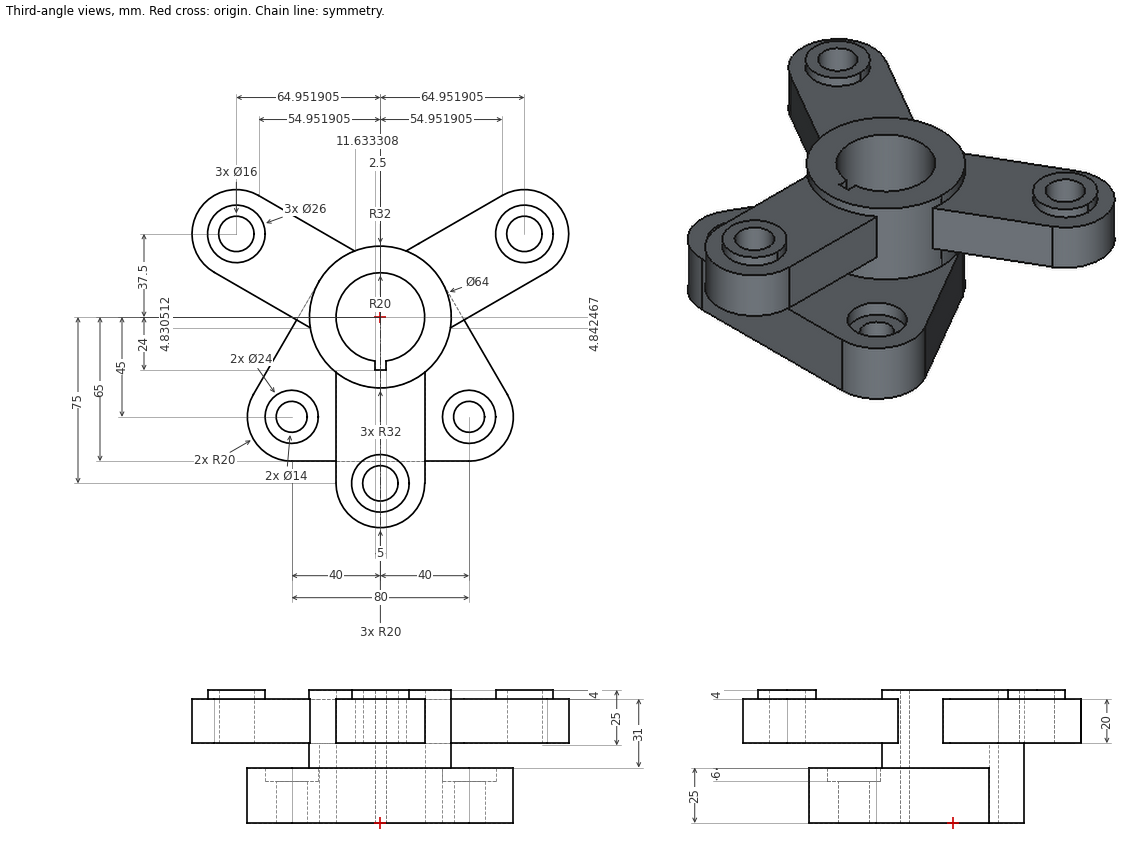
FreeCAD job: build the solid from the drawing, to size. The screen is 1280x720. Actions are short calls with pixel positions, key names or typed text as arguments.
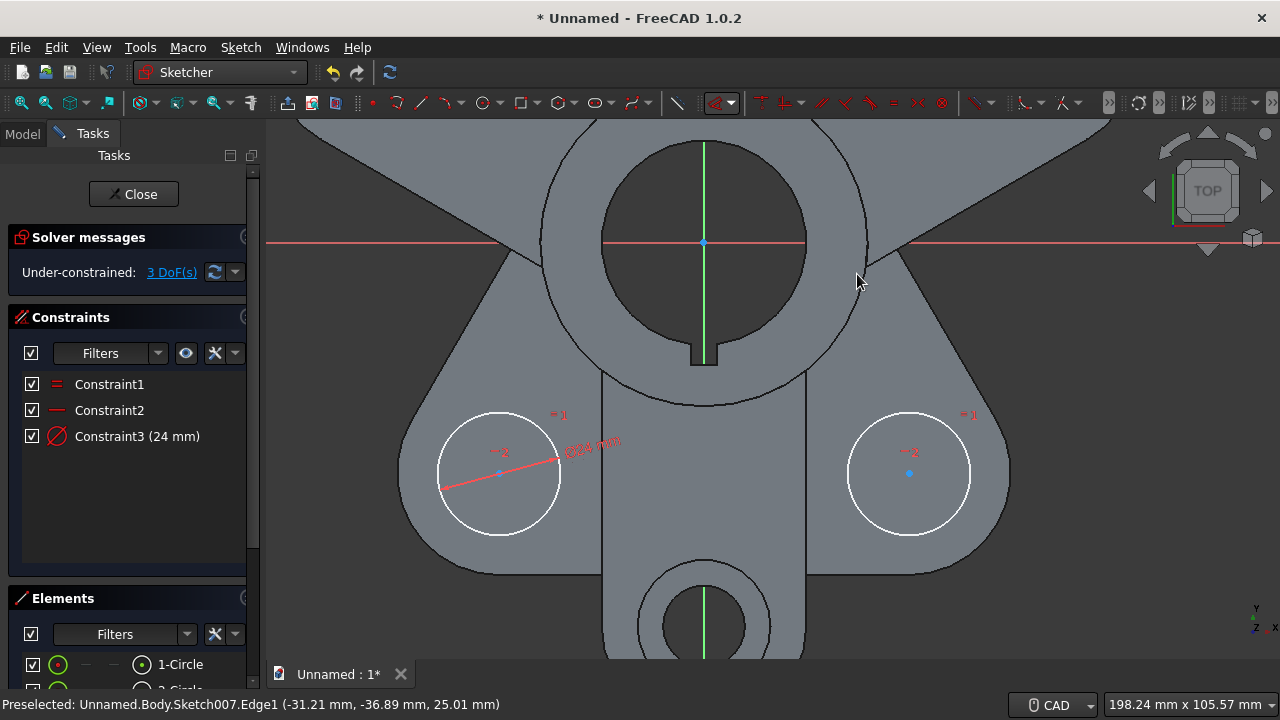
click(499, 474)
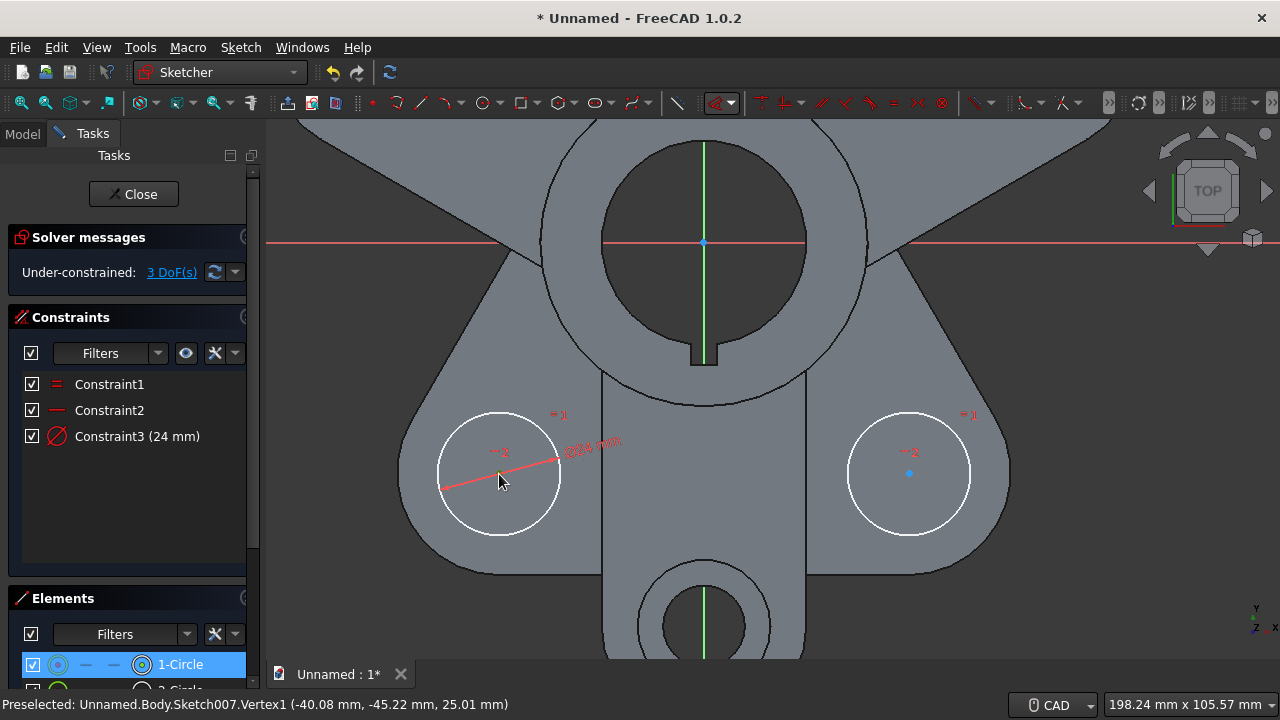
key(l)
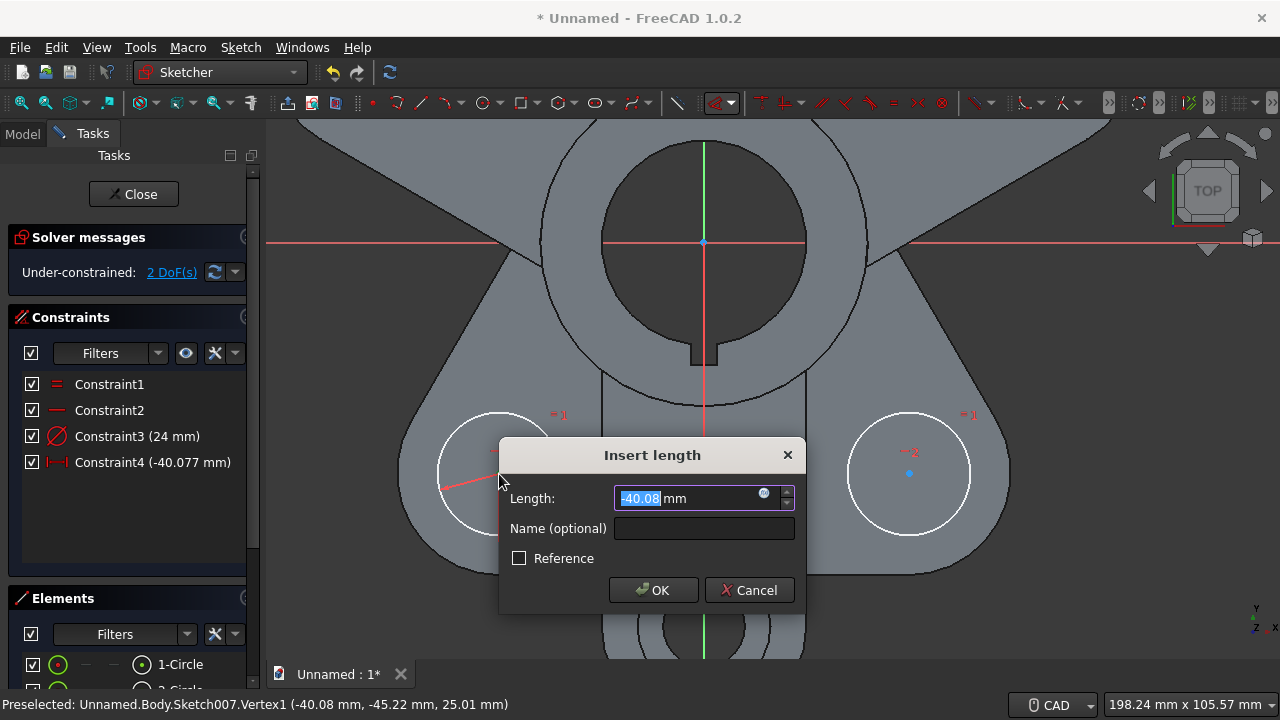
text(-40)
key(Return)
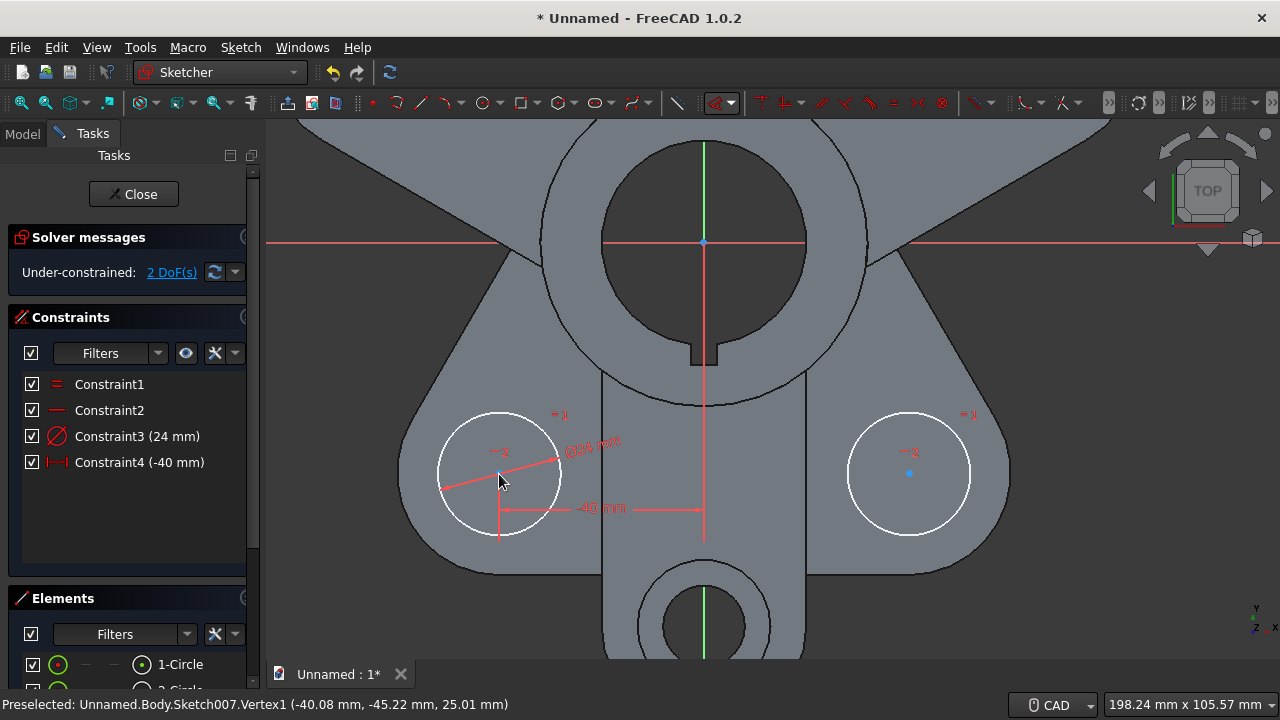
click(499, 474)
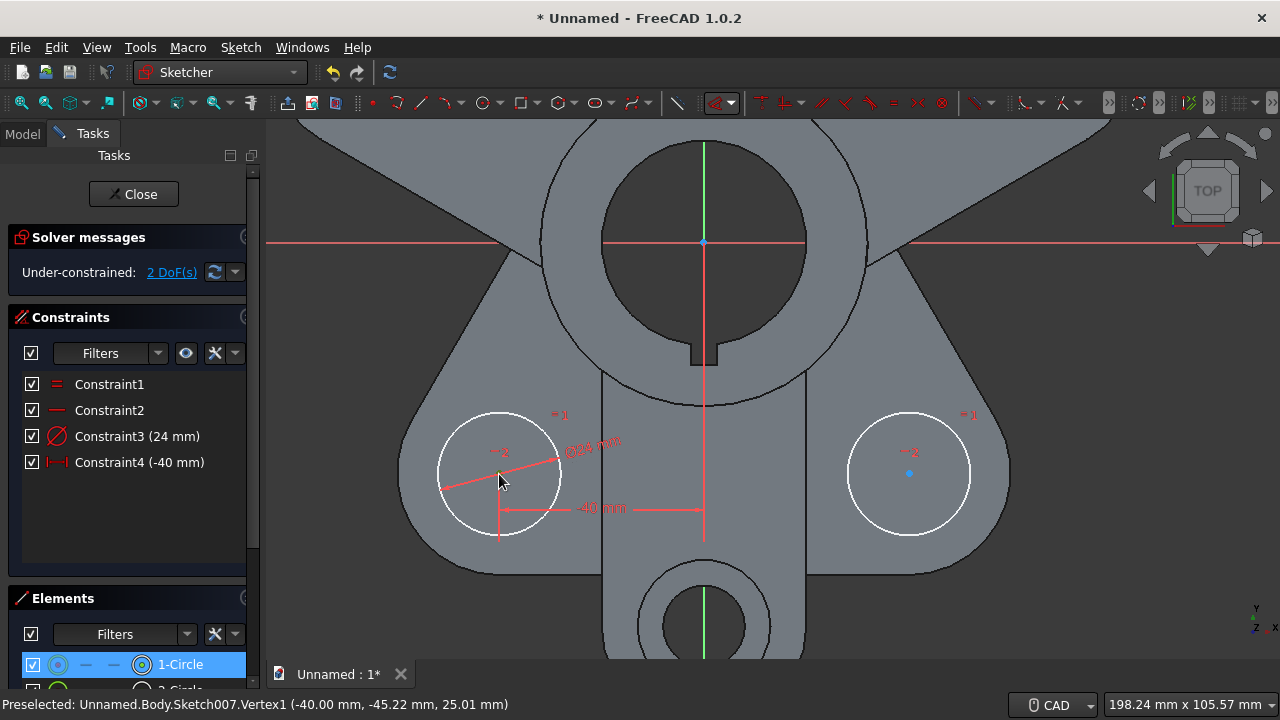
click(734, 104)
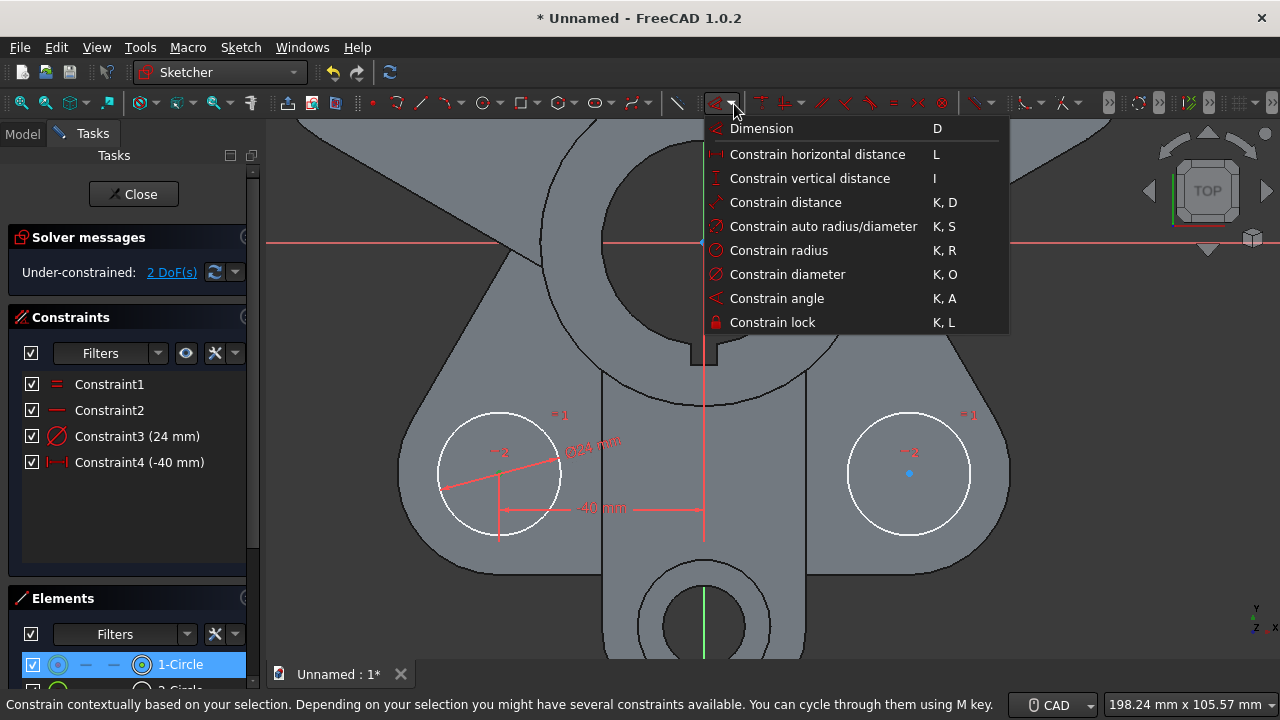
click(857, 178)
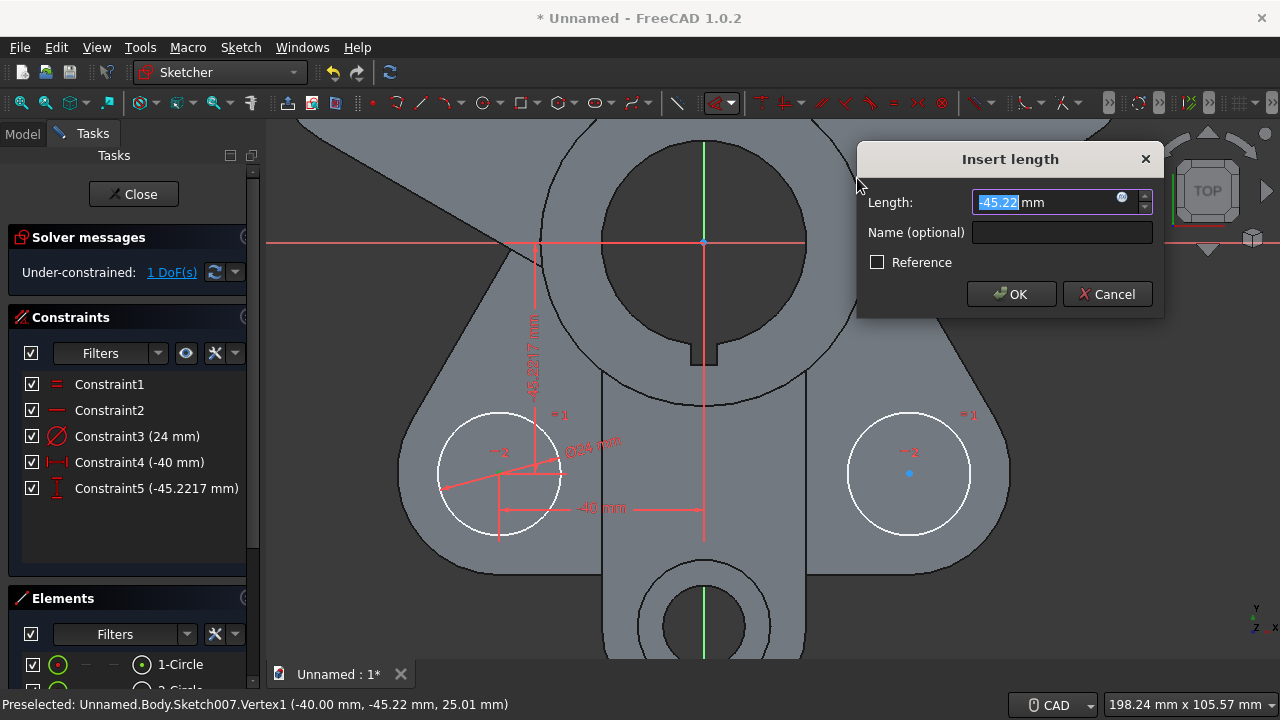
text(-45)
key(Return)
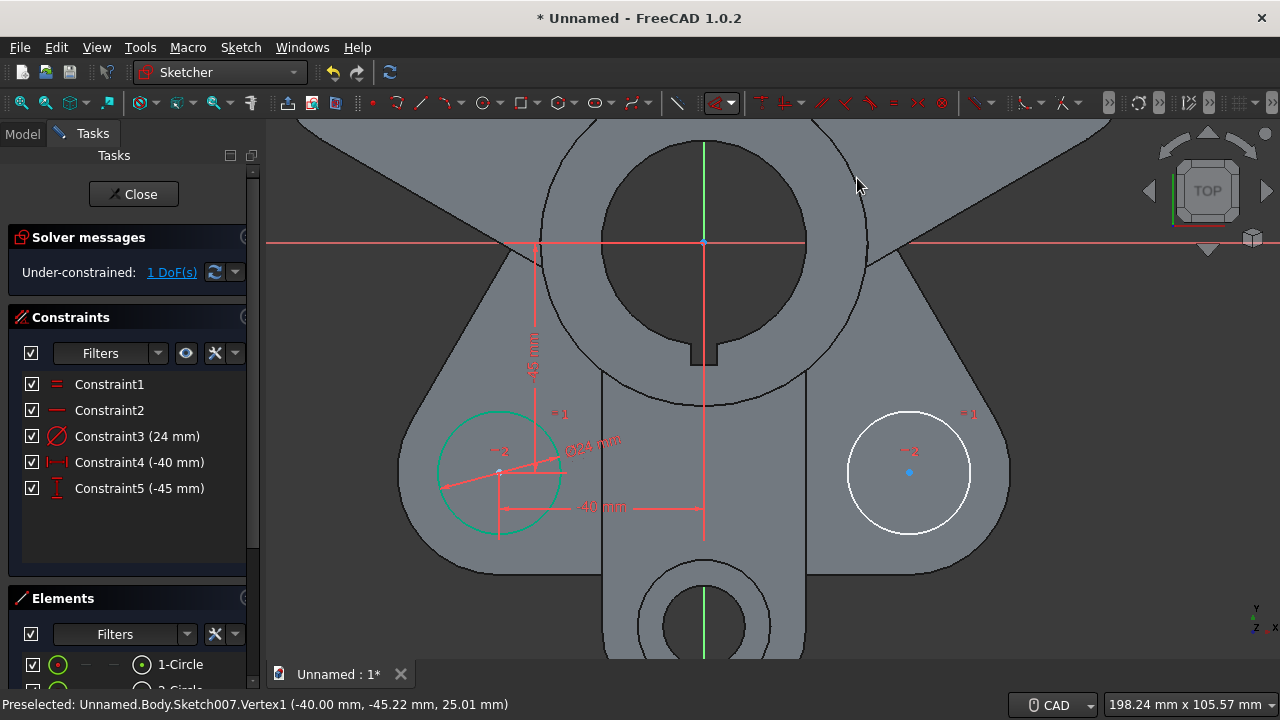
click(909, 473)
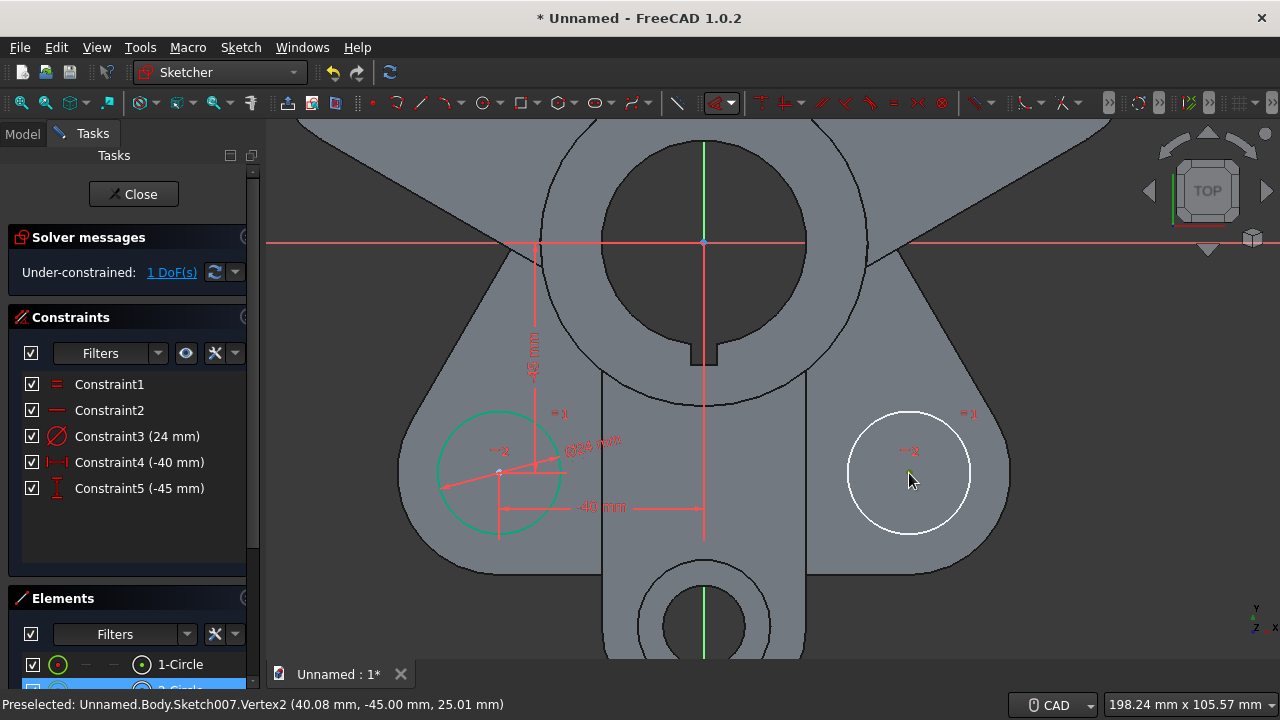
key(l)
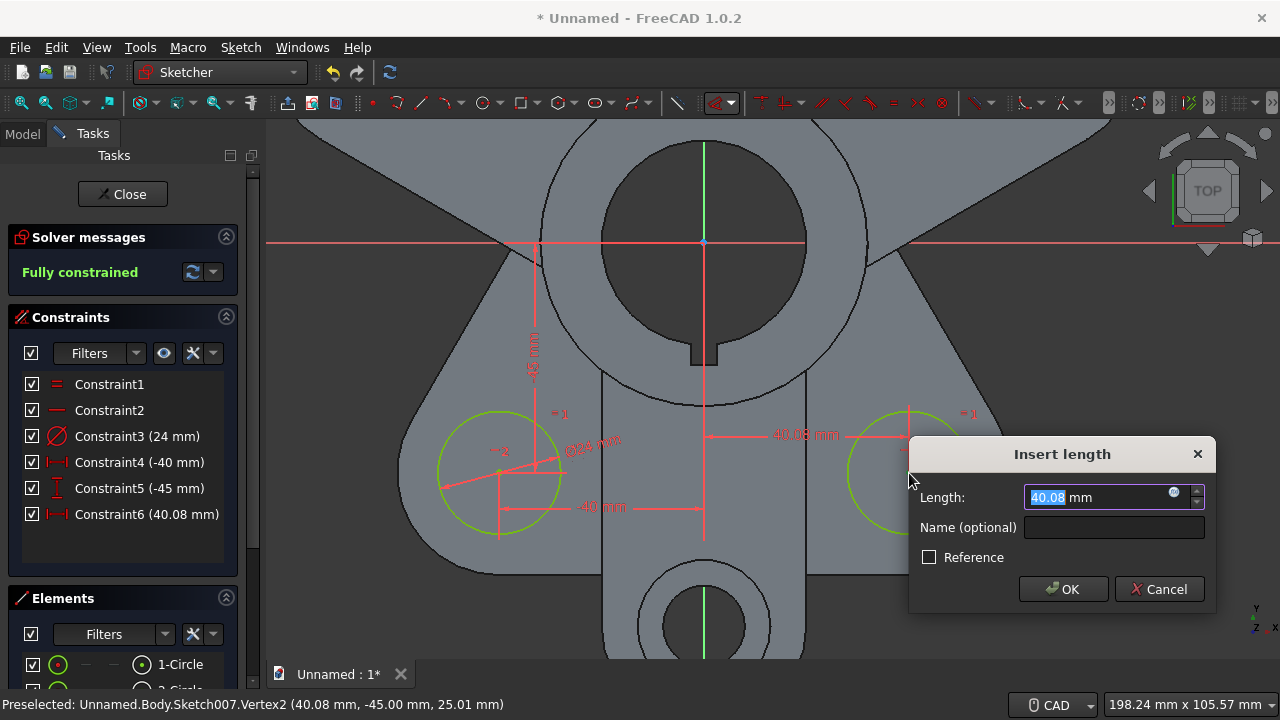
text(40)
key(Return)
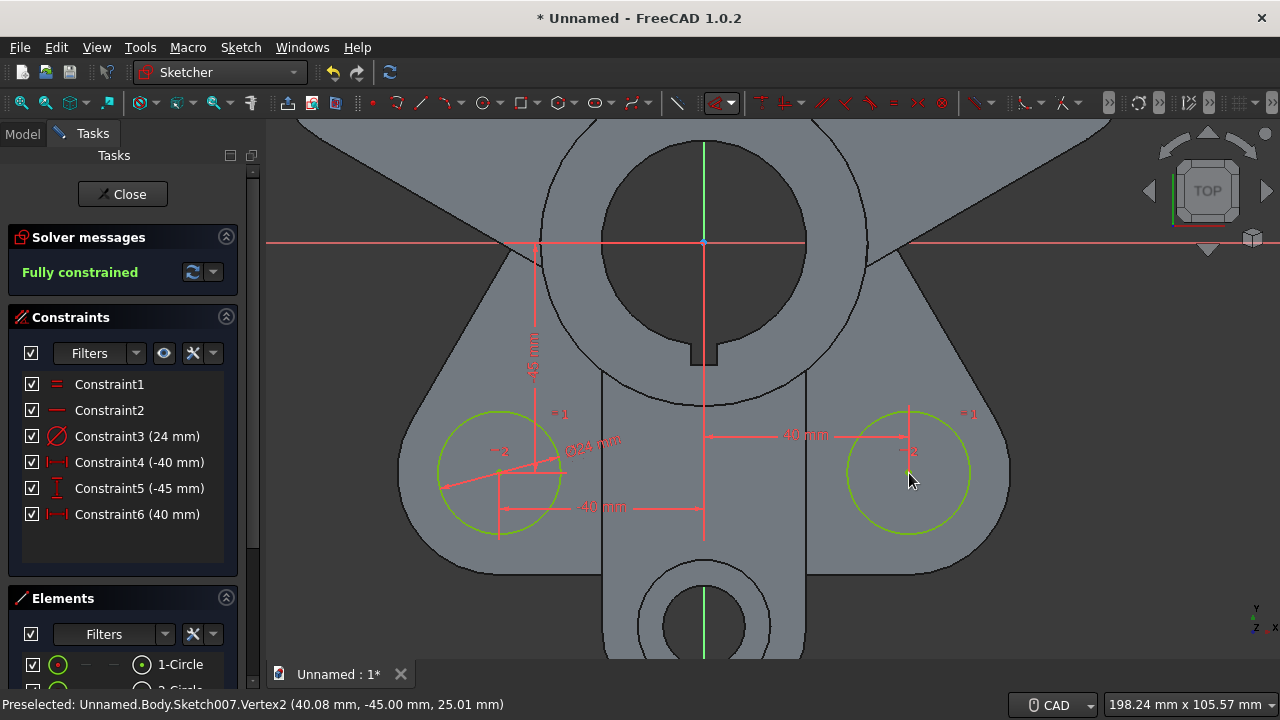
click(123, 194)